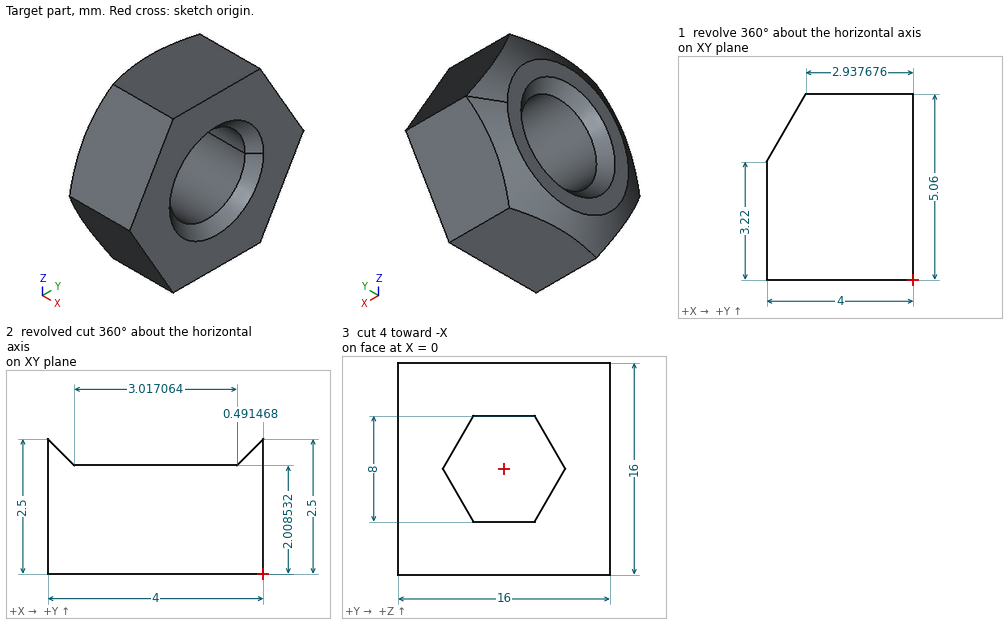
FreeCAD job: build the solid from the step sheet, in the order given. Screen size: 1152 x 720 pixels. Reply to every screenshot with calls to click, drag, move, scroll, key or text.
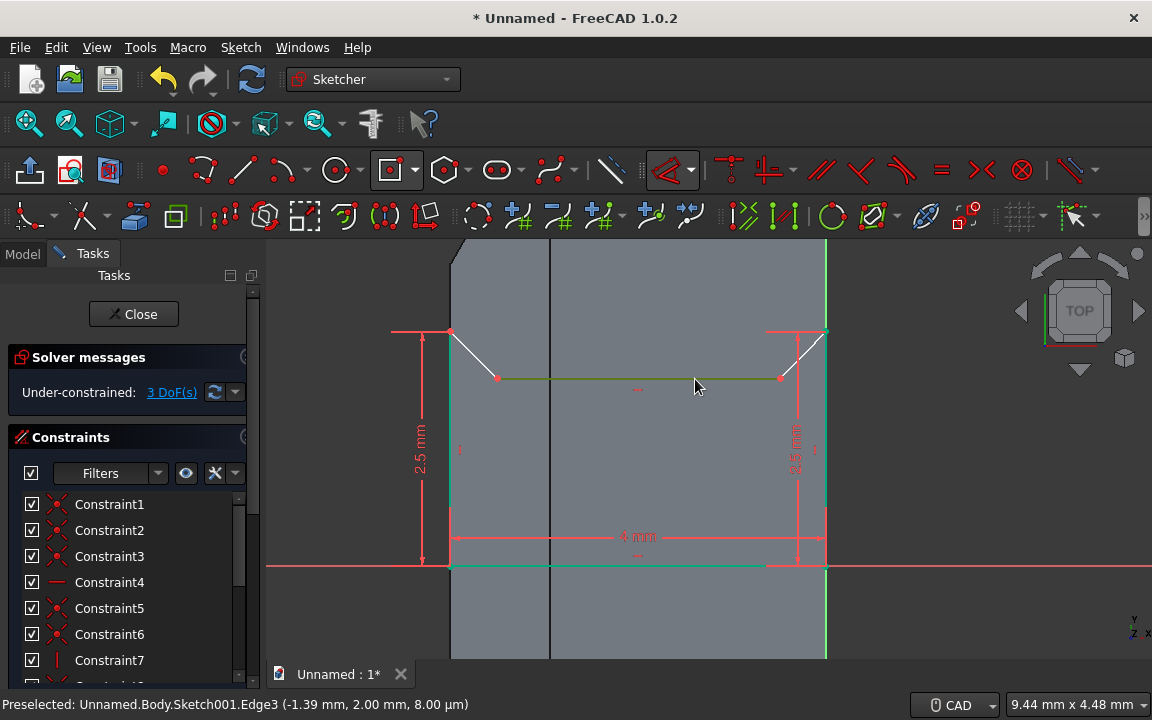
key(l)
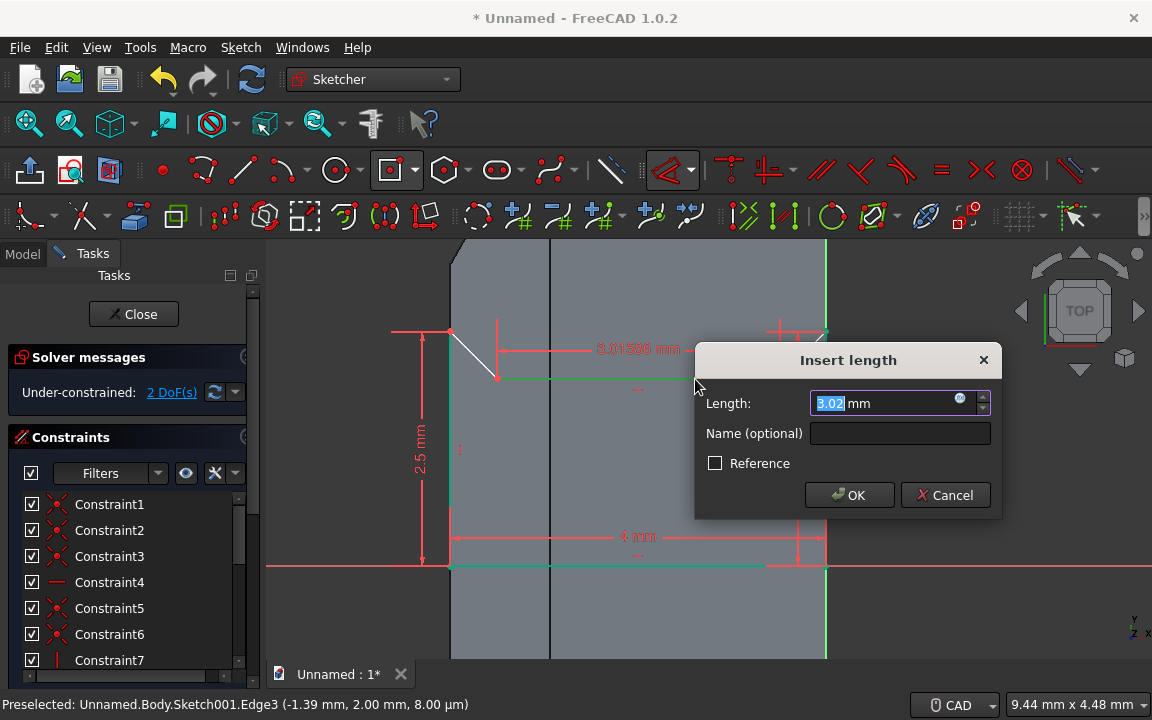
text(3.017064)
key(Return)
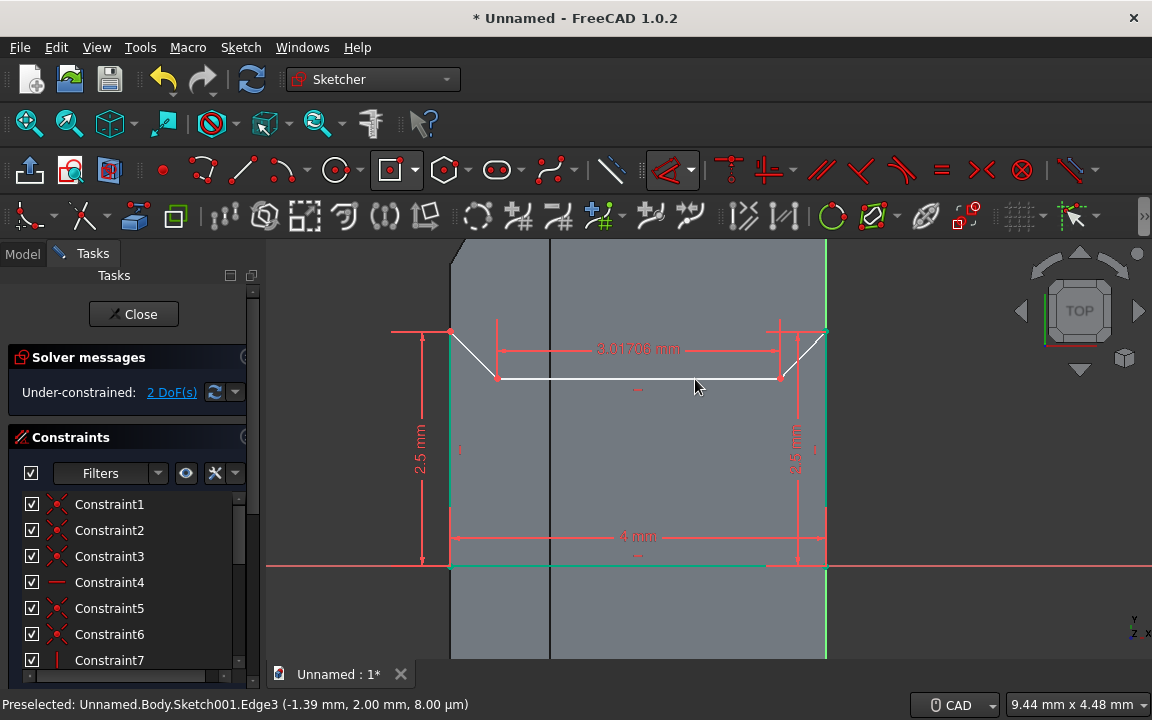
click(780, 379)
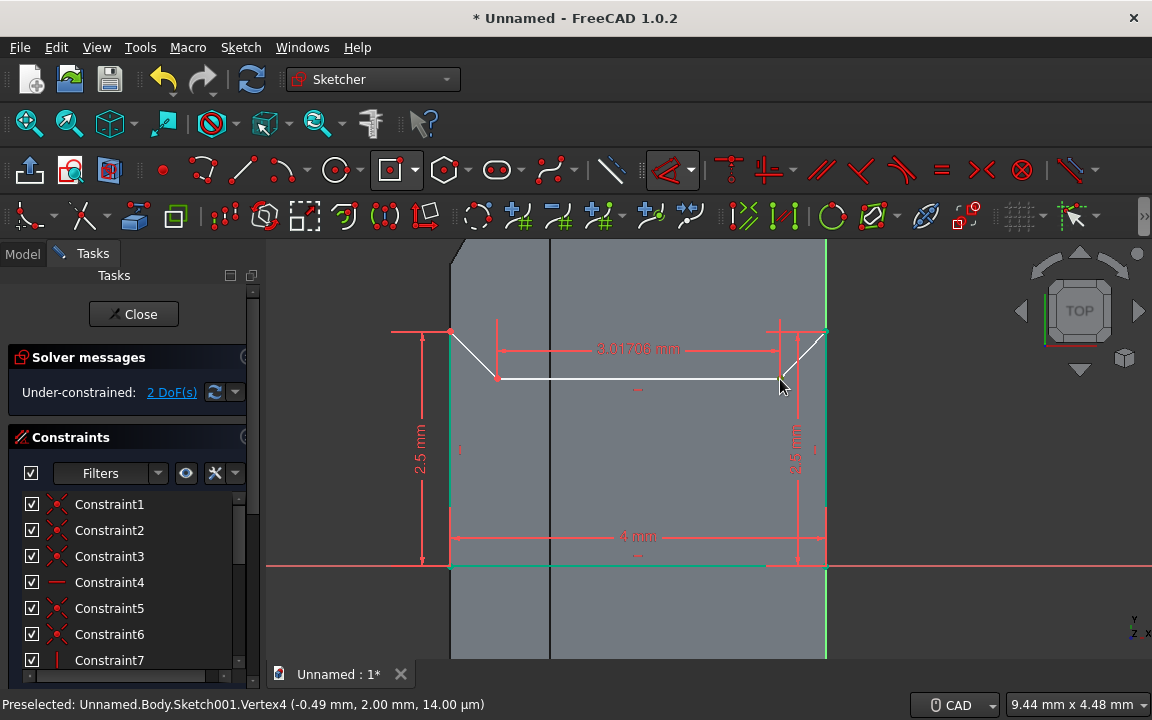
key(l)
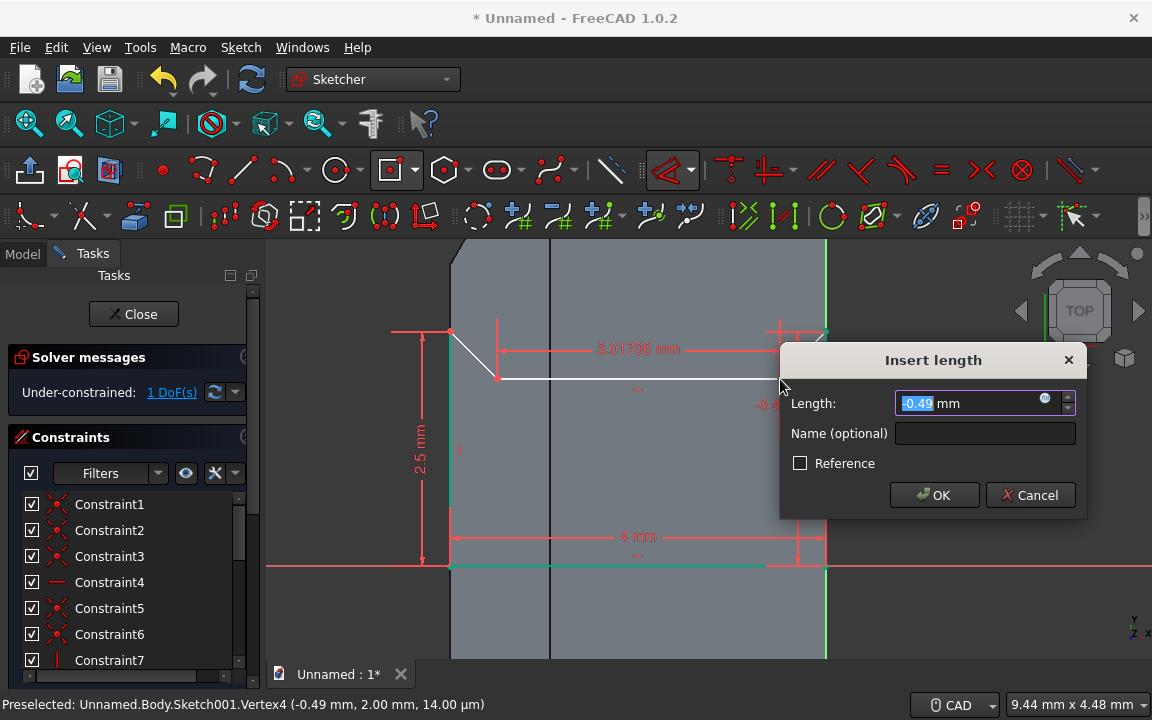
text(-0.491468)
key(Return)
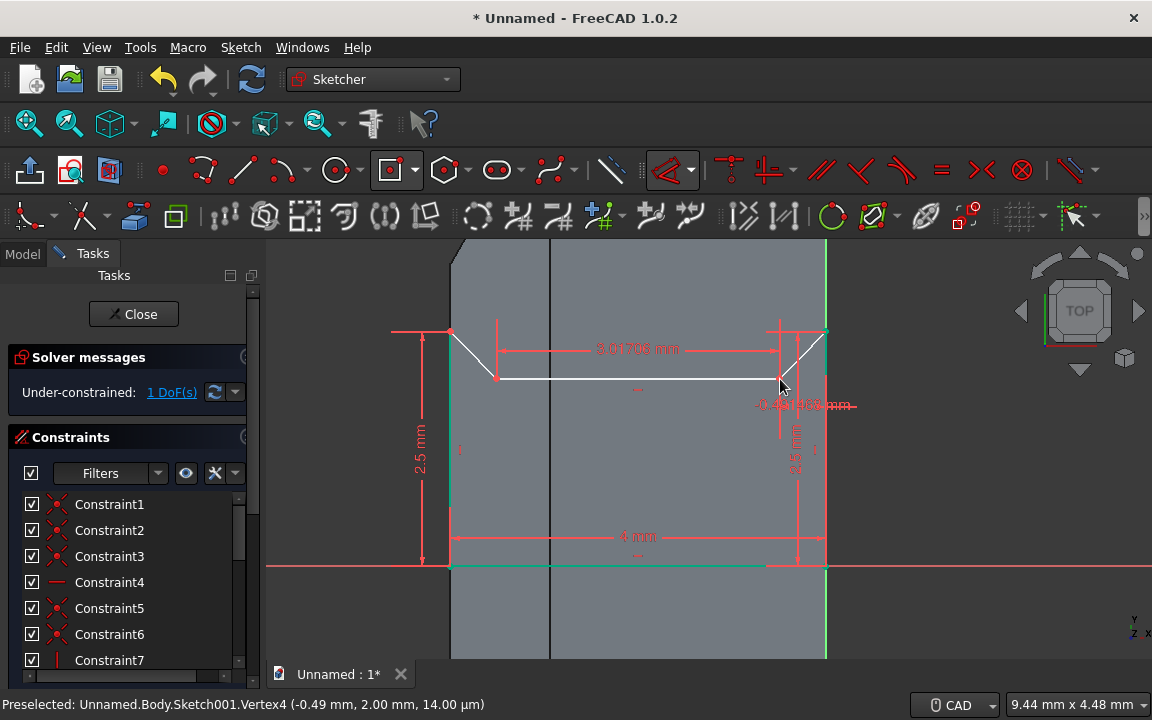
click(780, 379)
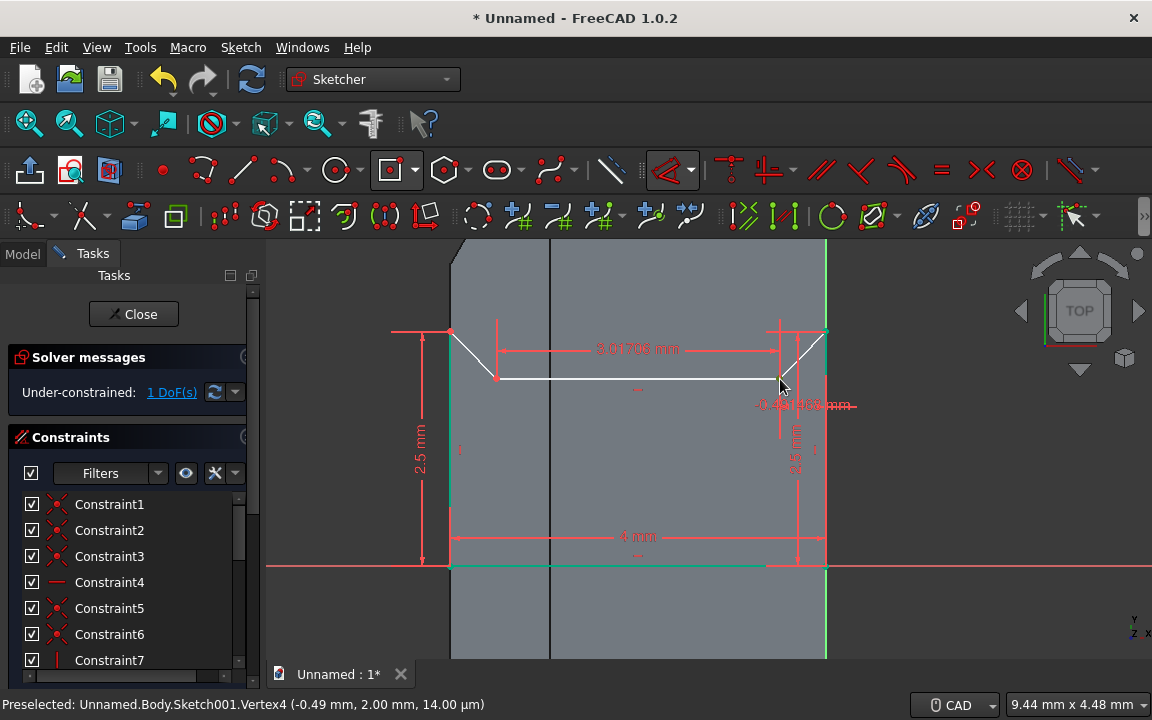
key(i)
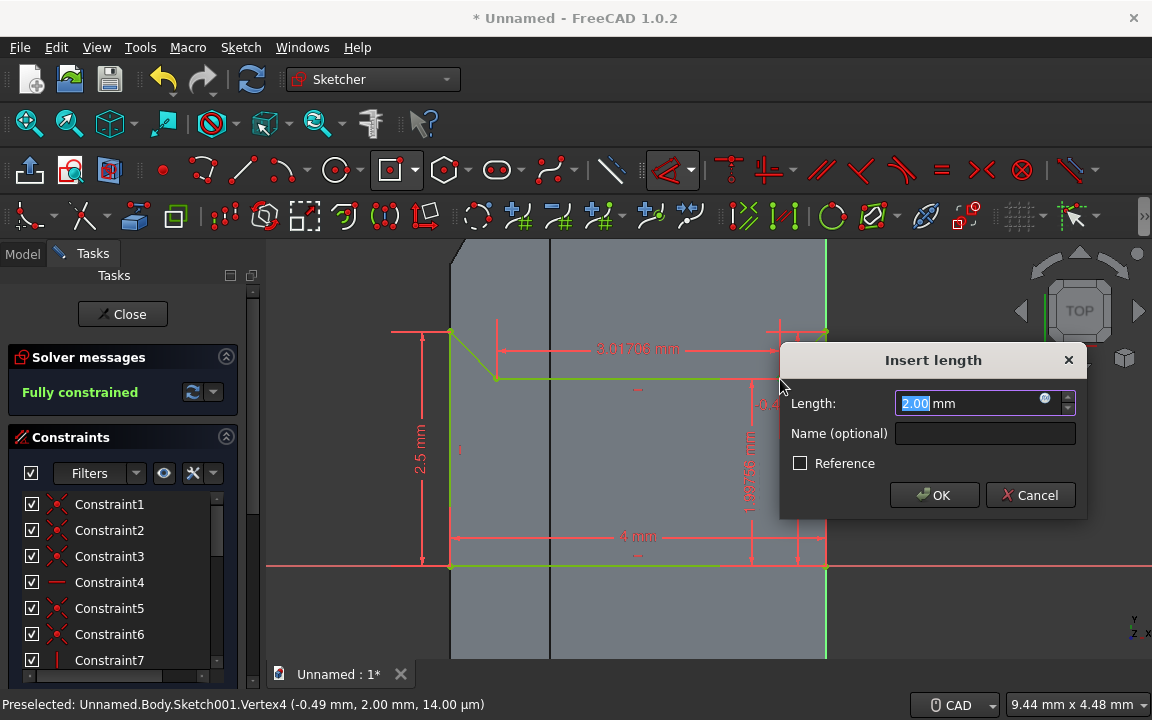
text(2.008532)
key(Return)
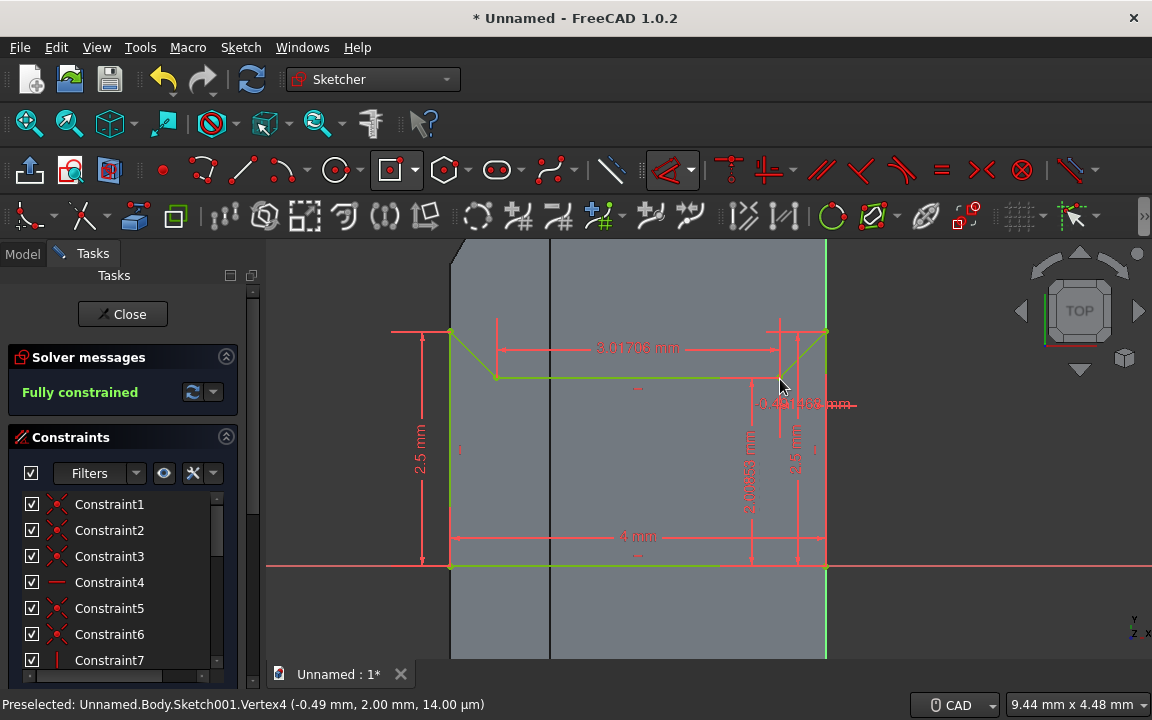
click(123, 314)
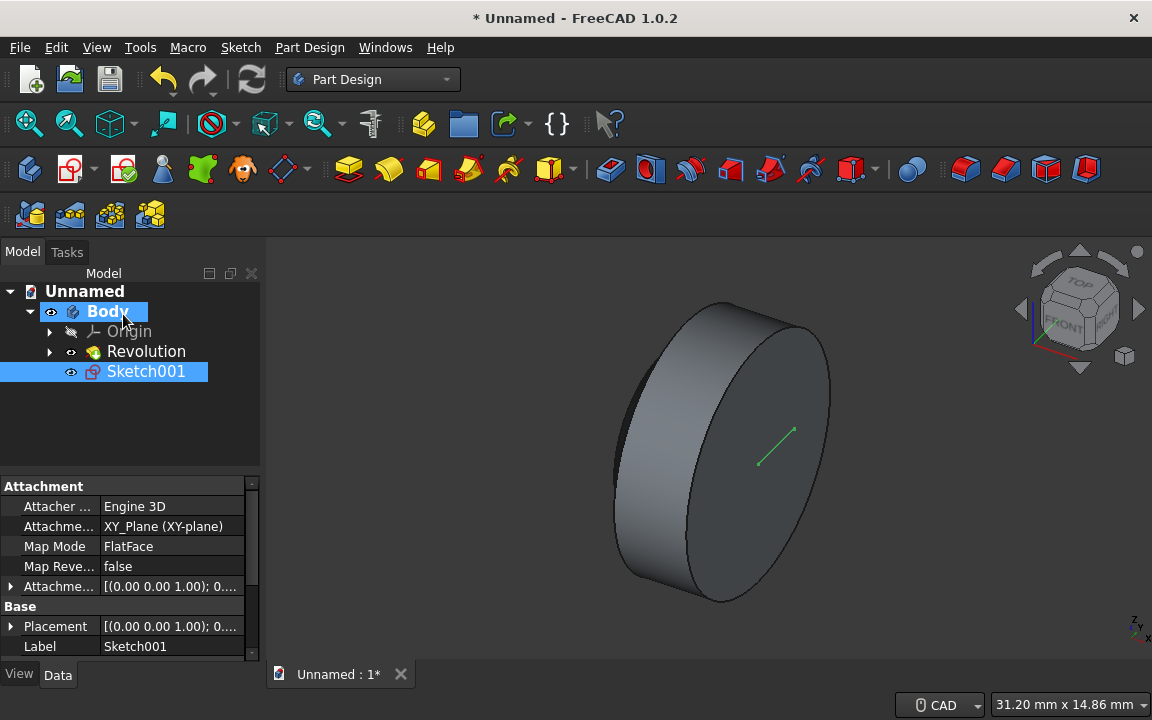
click(692, 170)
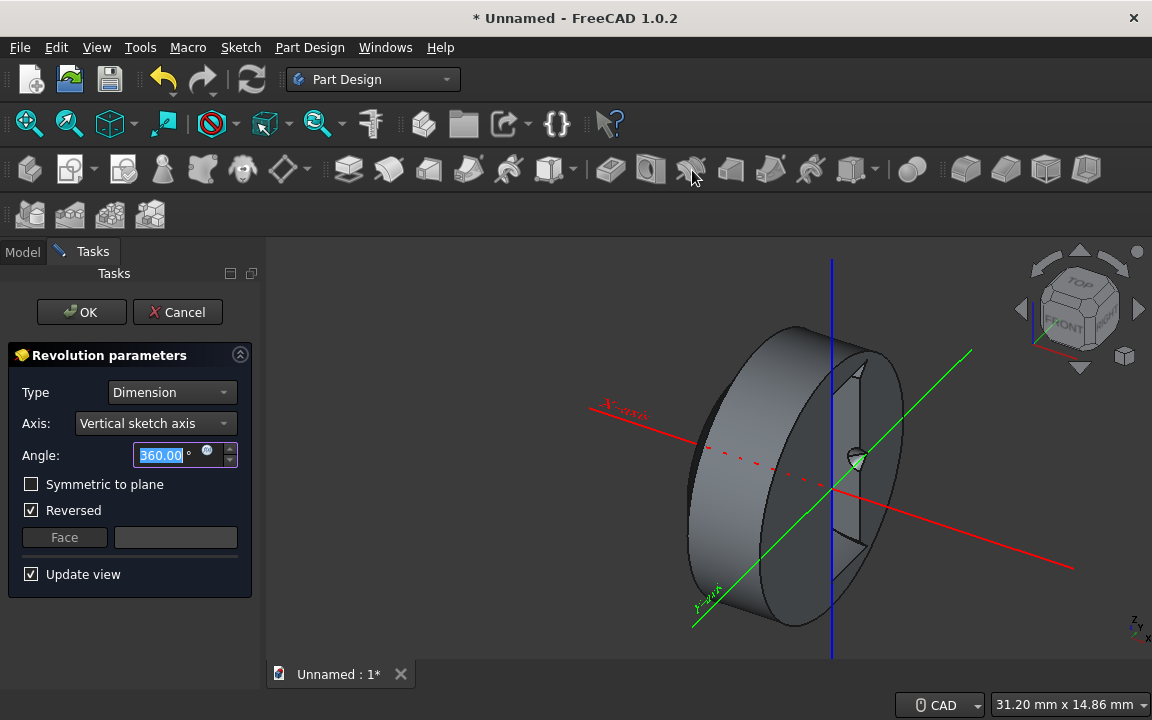
click(156, 424)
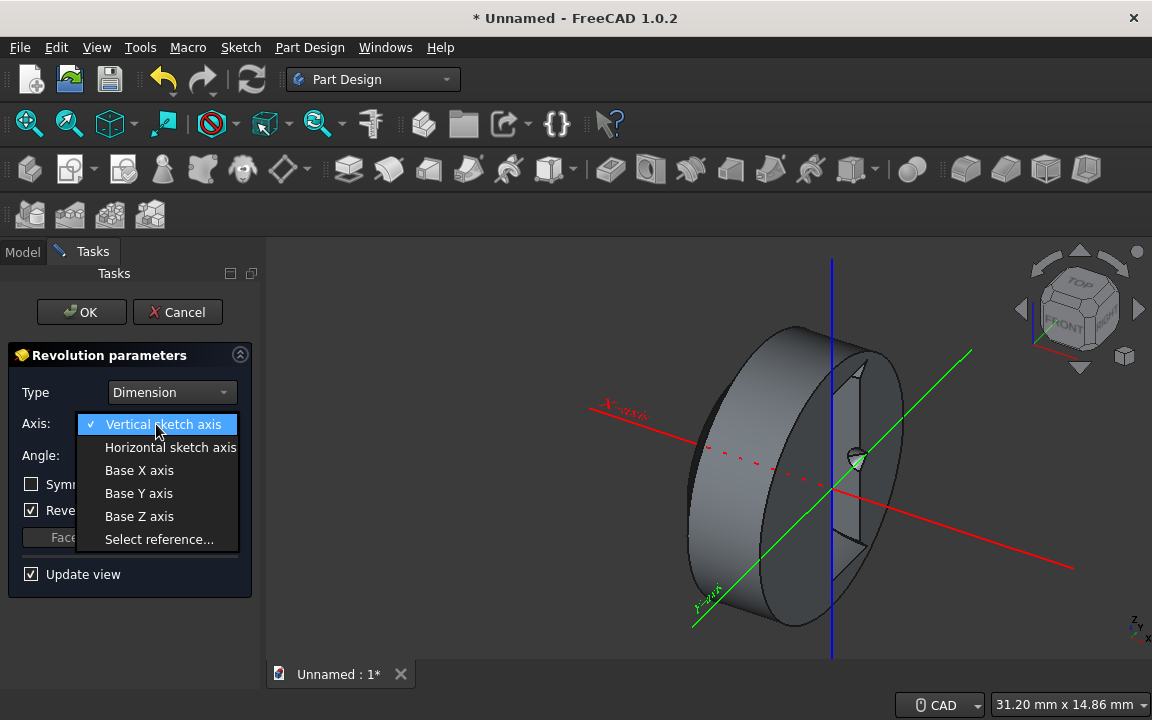
click(156, 448)